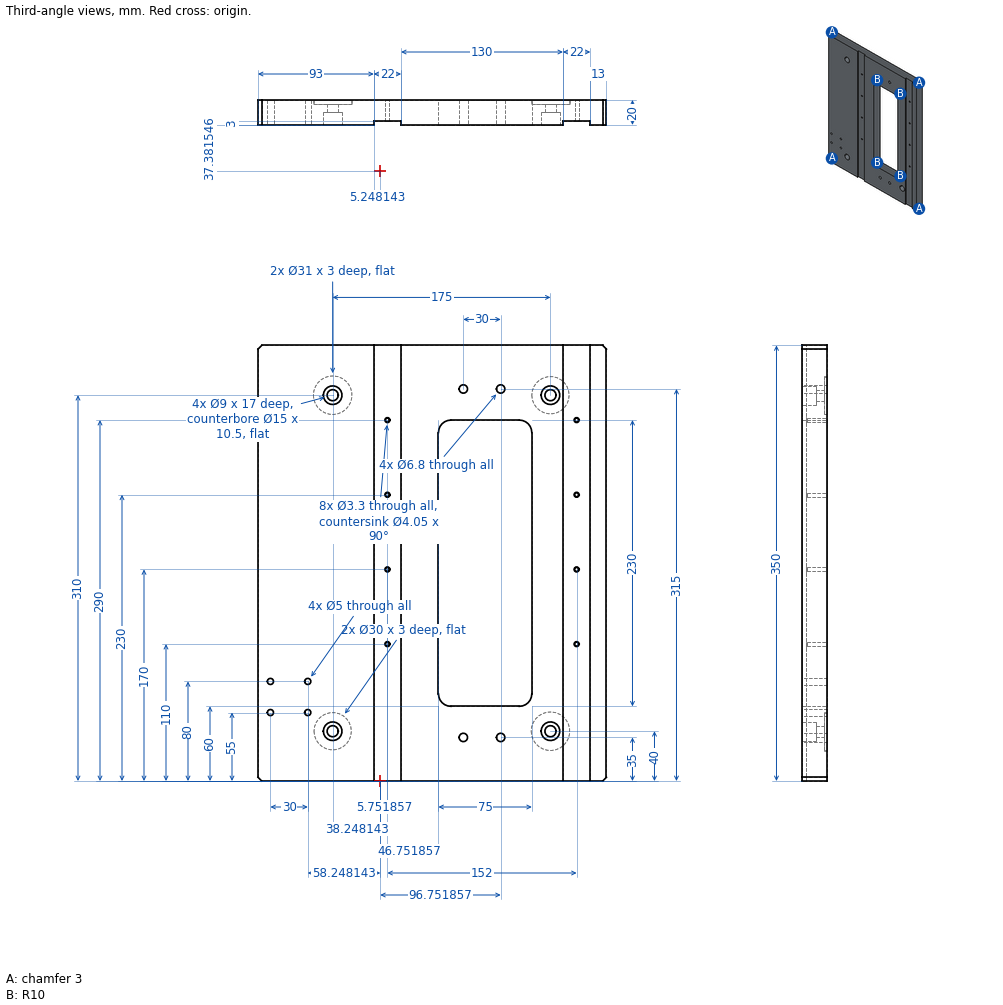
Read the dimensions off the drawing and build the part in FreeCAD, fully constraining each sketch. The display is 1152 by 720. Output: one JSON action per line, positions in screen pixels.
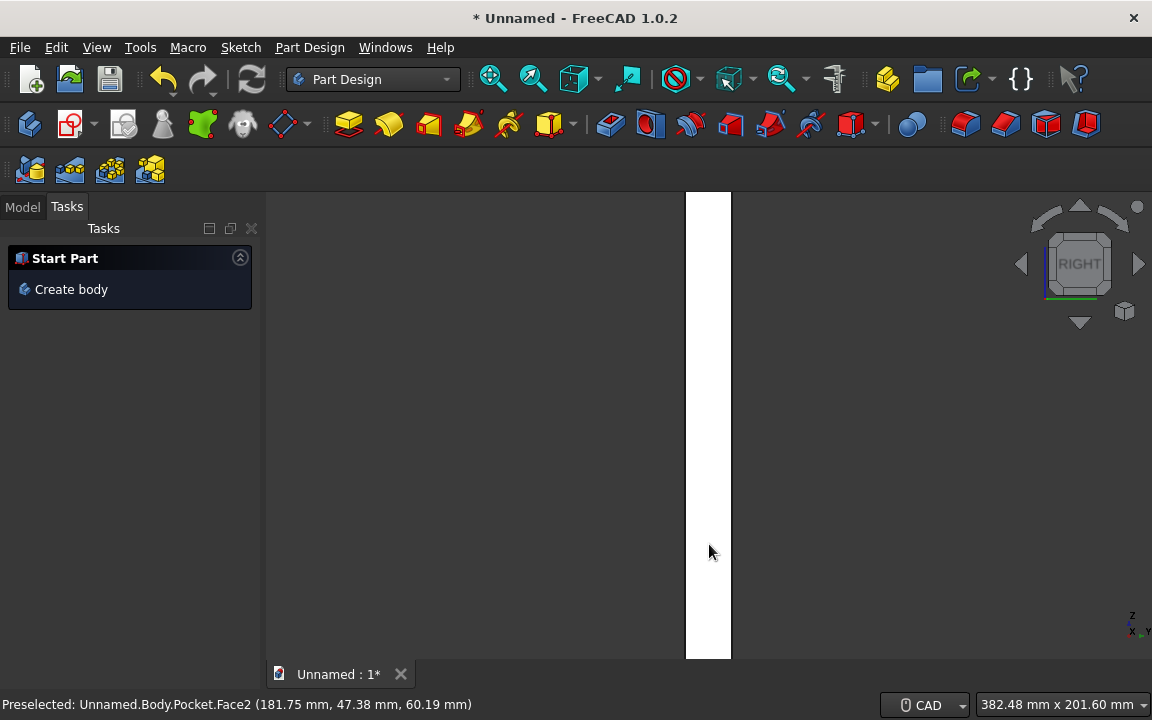
{"action": "left_click", "coordinate": [494, 80]}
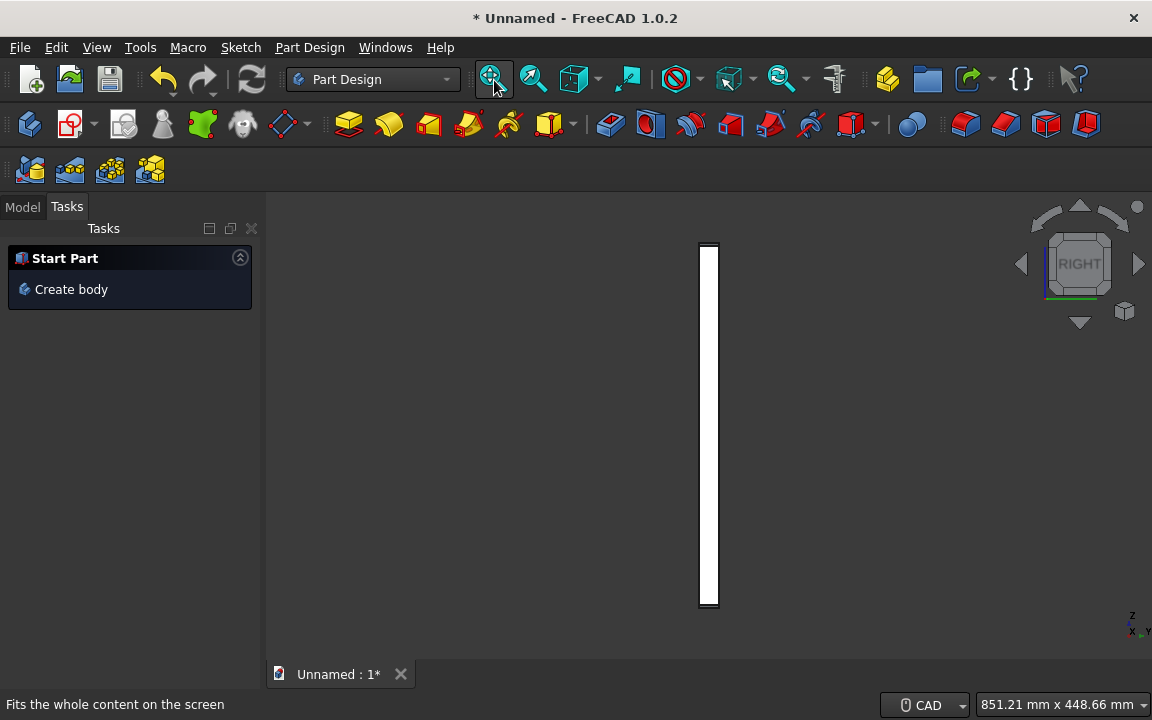
{"action": "key", "text": "5"}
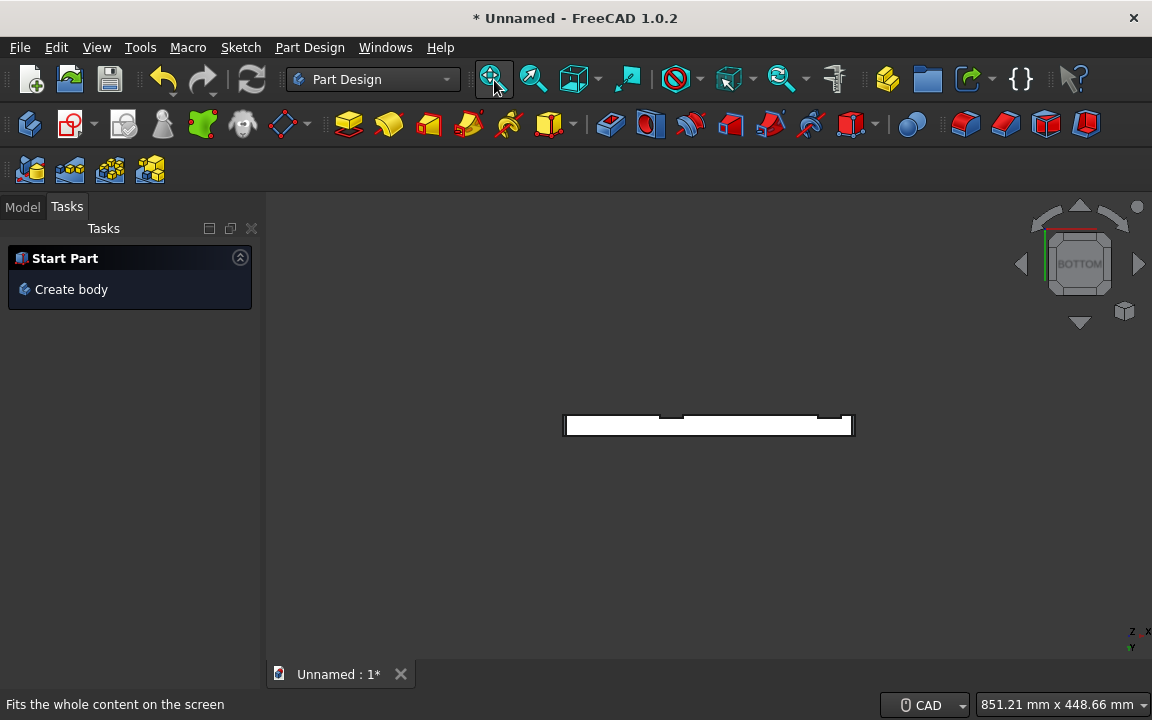
{"action": "left_click", "coordinate": [494, 80]}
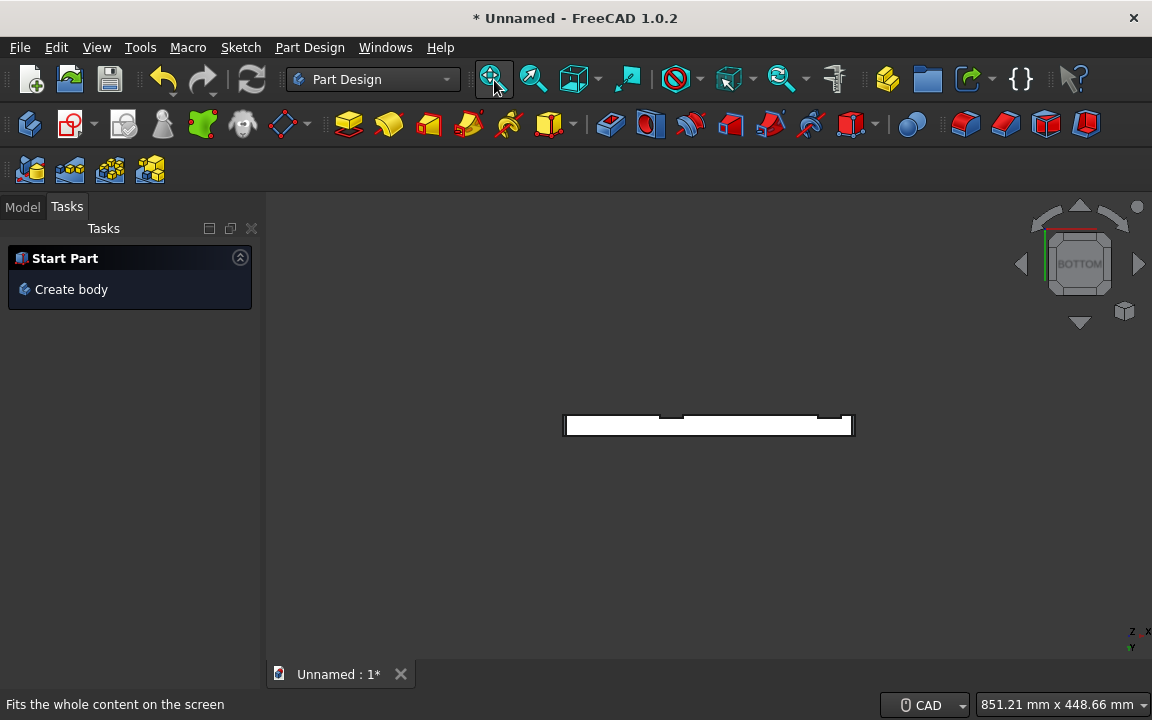
{"action": "scroll", "coordinate": [714, 424], "scroll_direction": "up", "scroll_amount": 4}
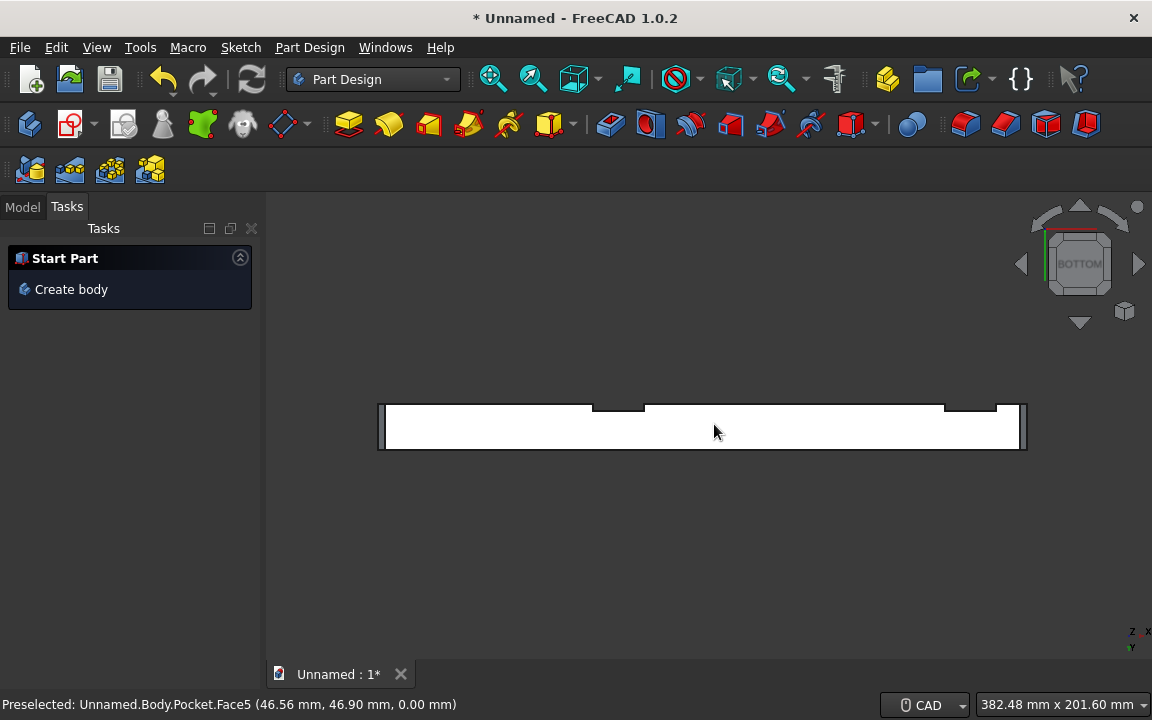
{"action": "left_click", "coordinate": [494, 80]}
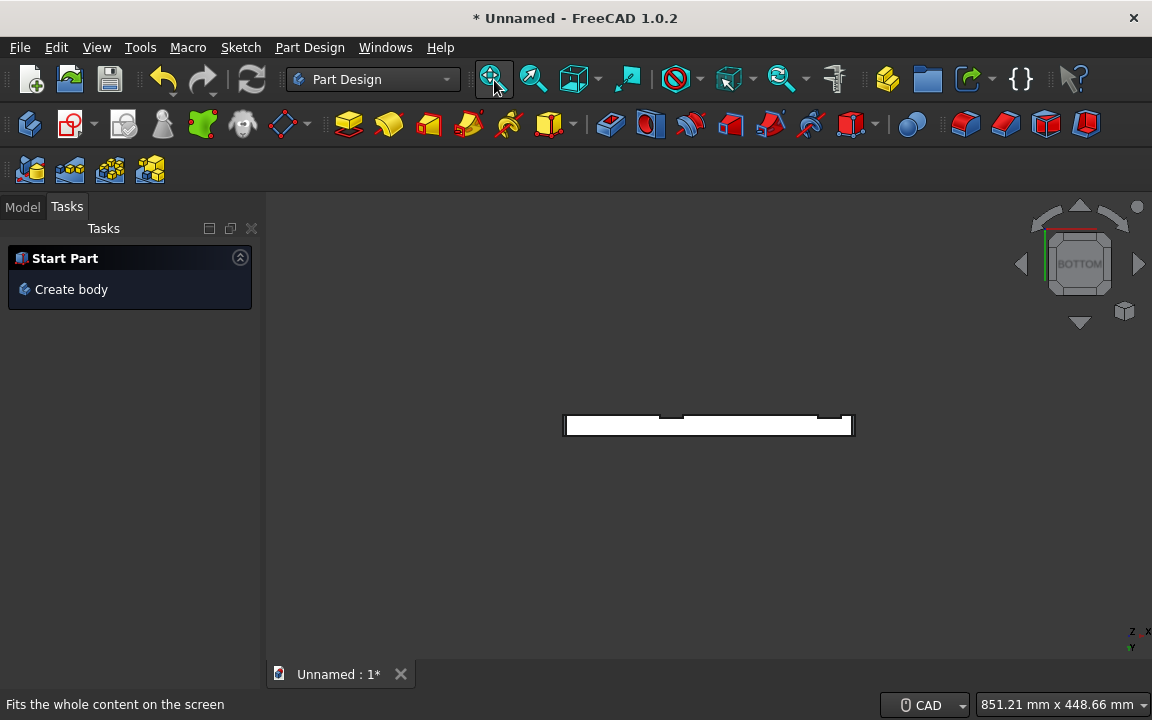
{"action": "key", "text": "4"}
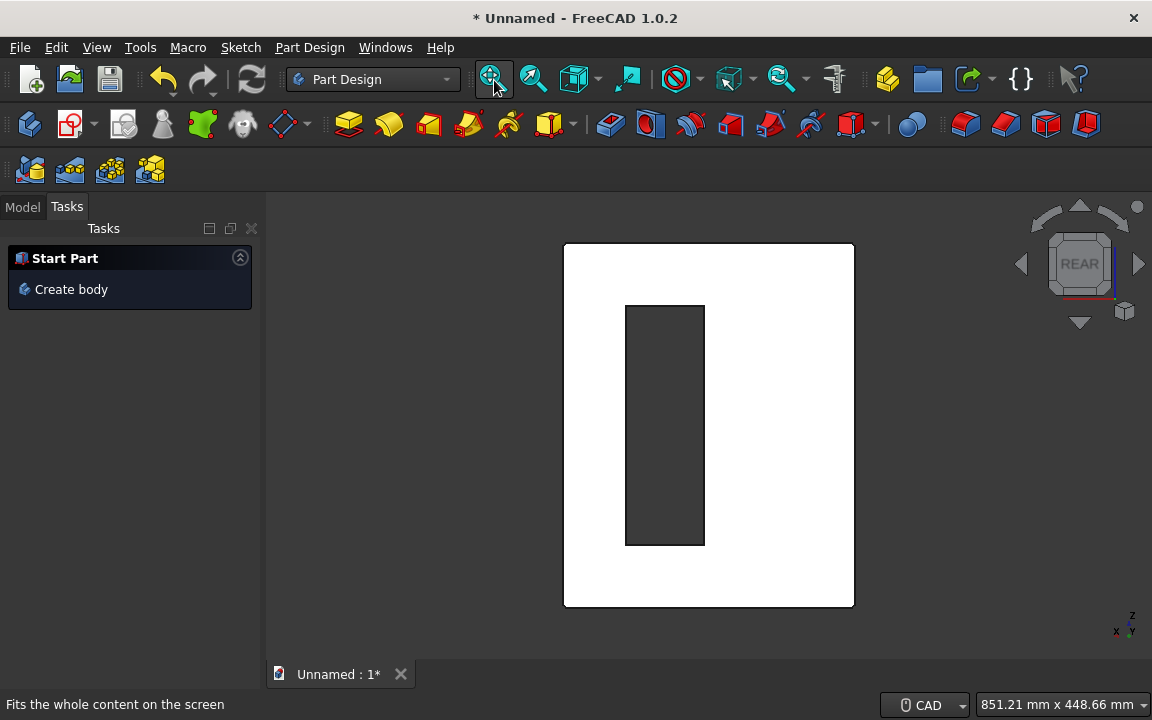
{"action": "scroll", "coordinate": [704, 544], "scroll_direction": "up", "scroll_amount": 4}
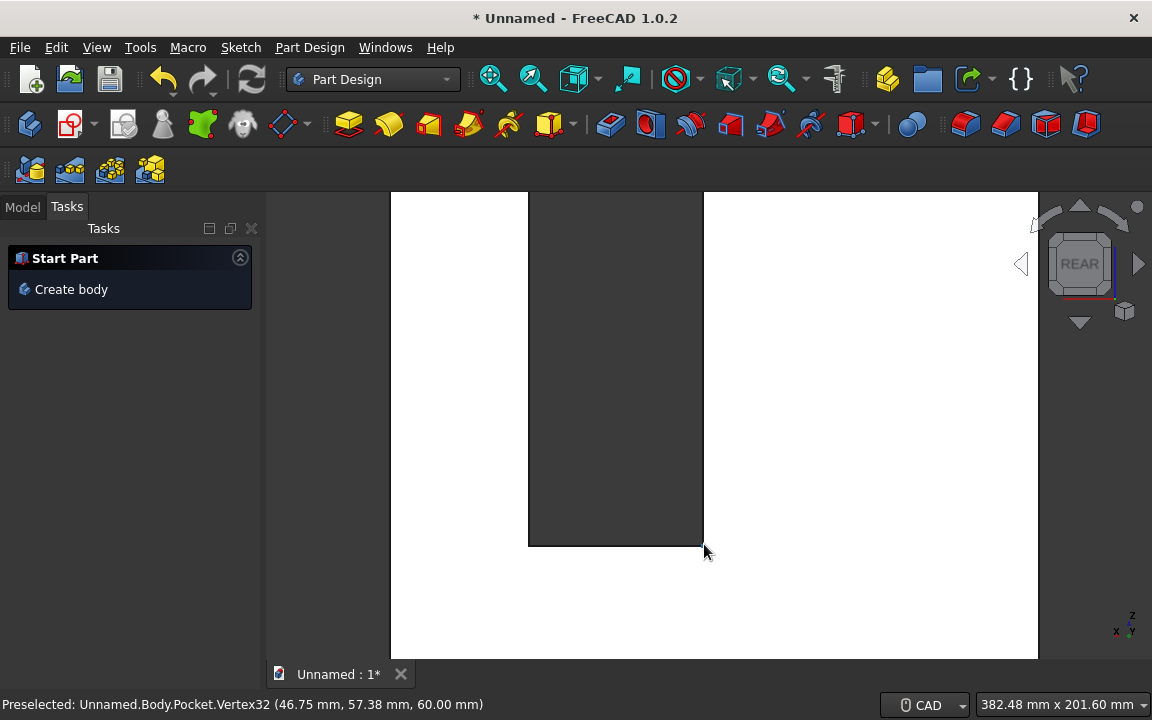
{"action": "left_click", "coordinate": [494, 80]}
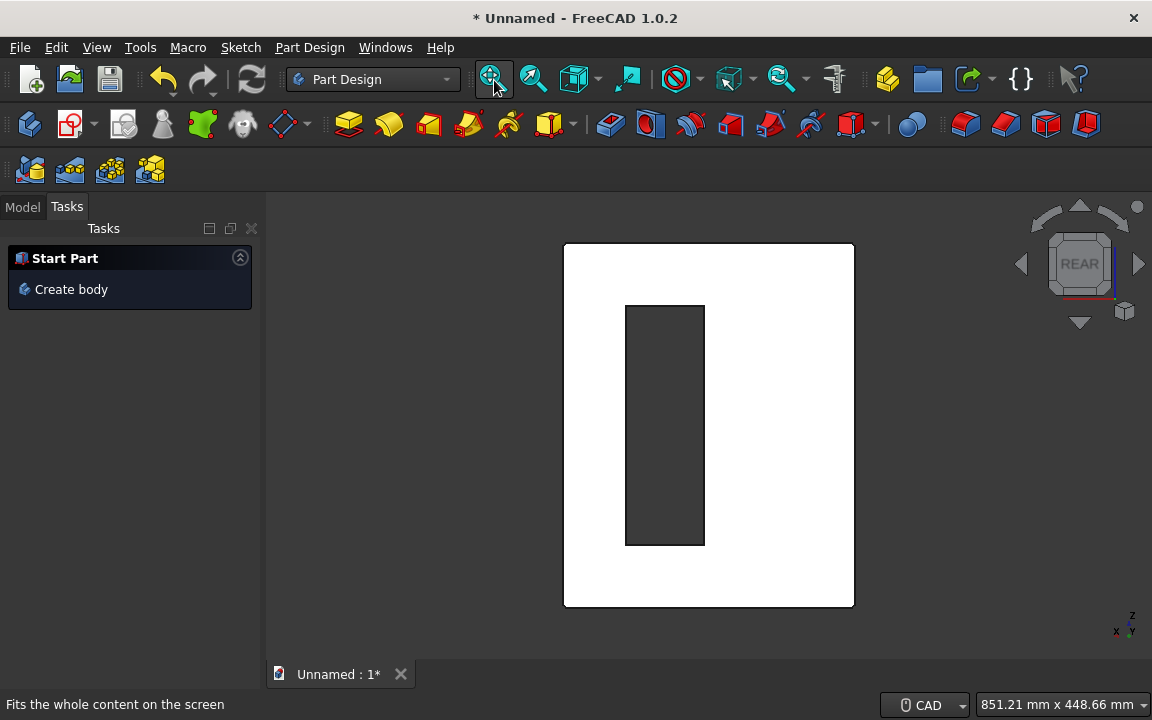
{"action": "key", "text": "6"}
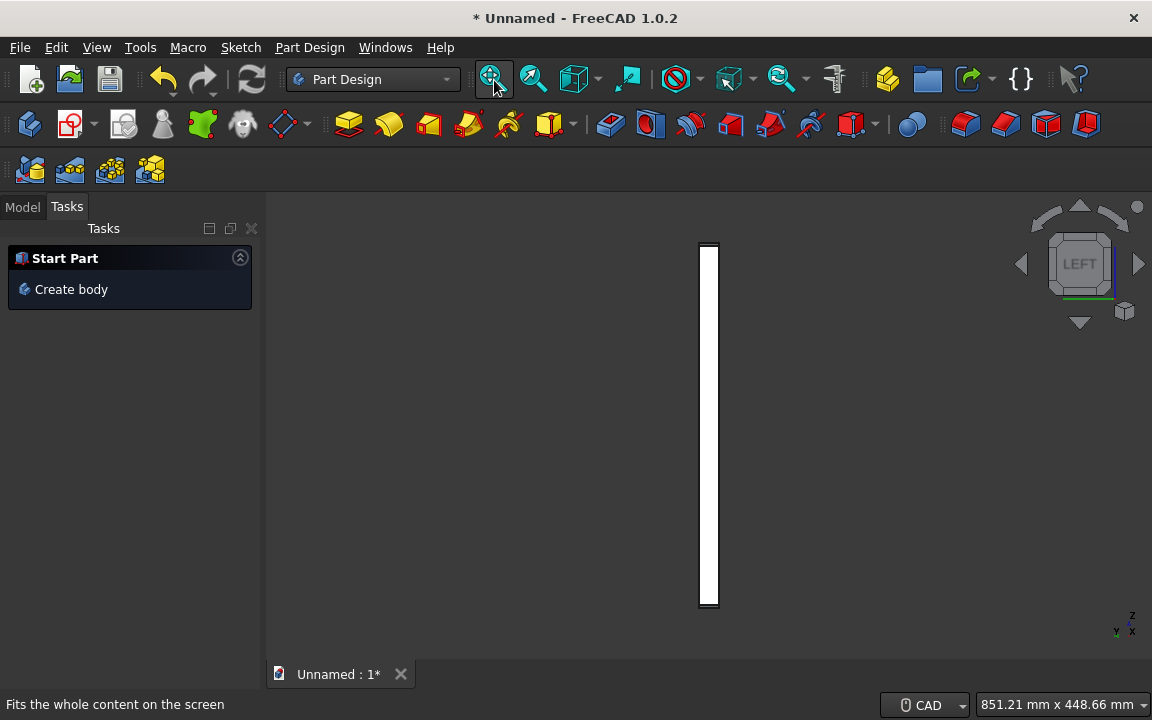
{"action": "scroll", "coordinate": [709, 544], "scroll_direction": "up", "scroll_amount": 4}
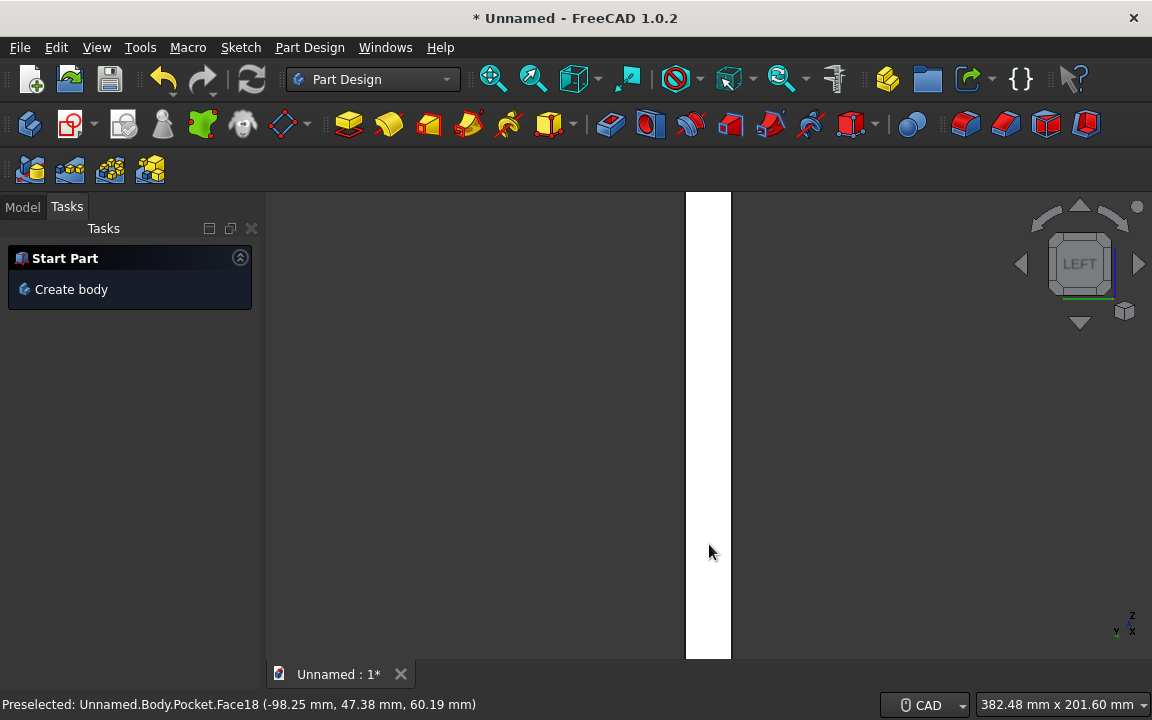
{"action": "left_click", "coordinate": [494, 80]}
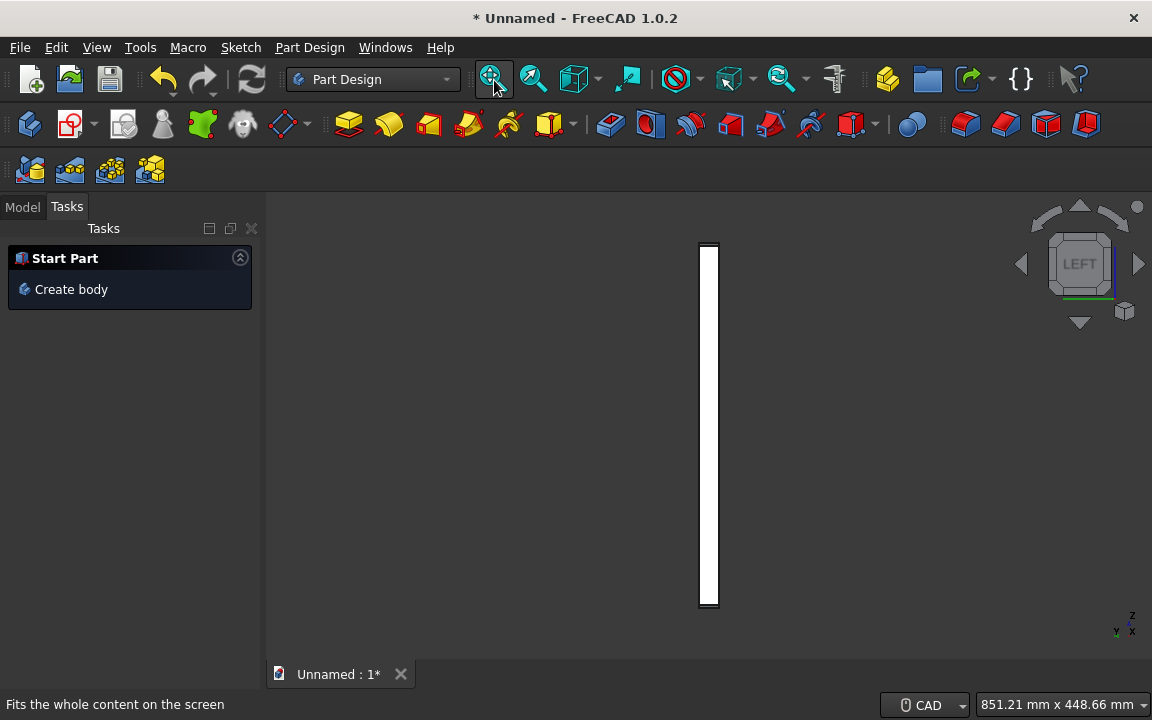
{"action": "key", "text": "v 3"}